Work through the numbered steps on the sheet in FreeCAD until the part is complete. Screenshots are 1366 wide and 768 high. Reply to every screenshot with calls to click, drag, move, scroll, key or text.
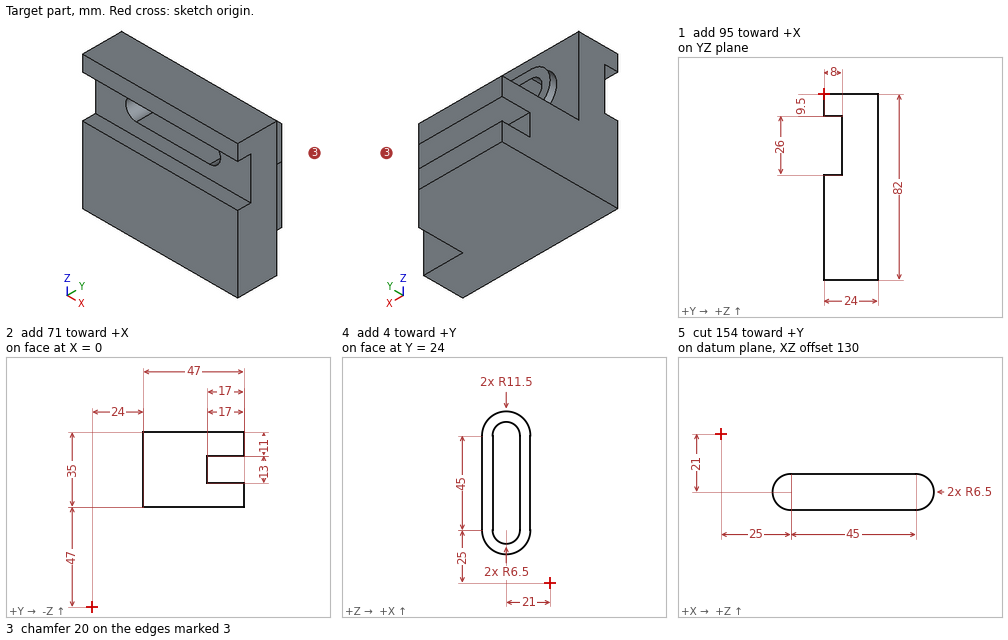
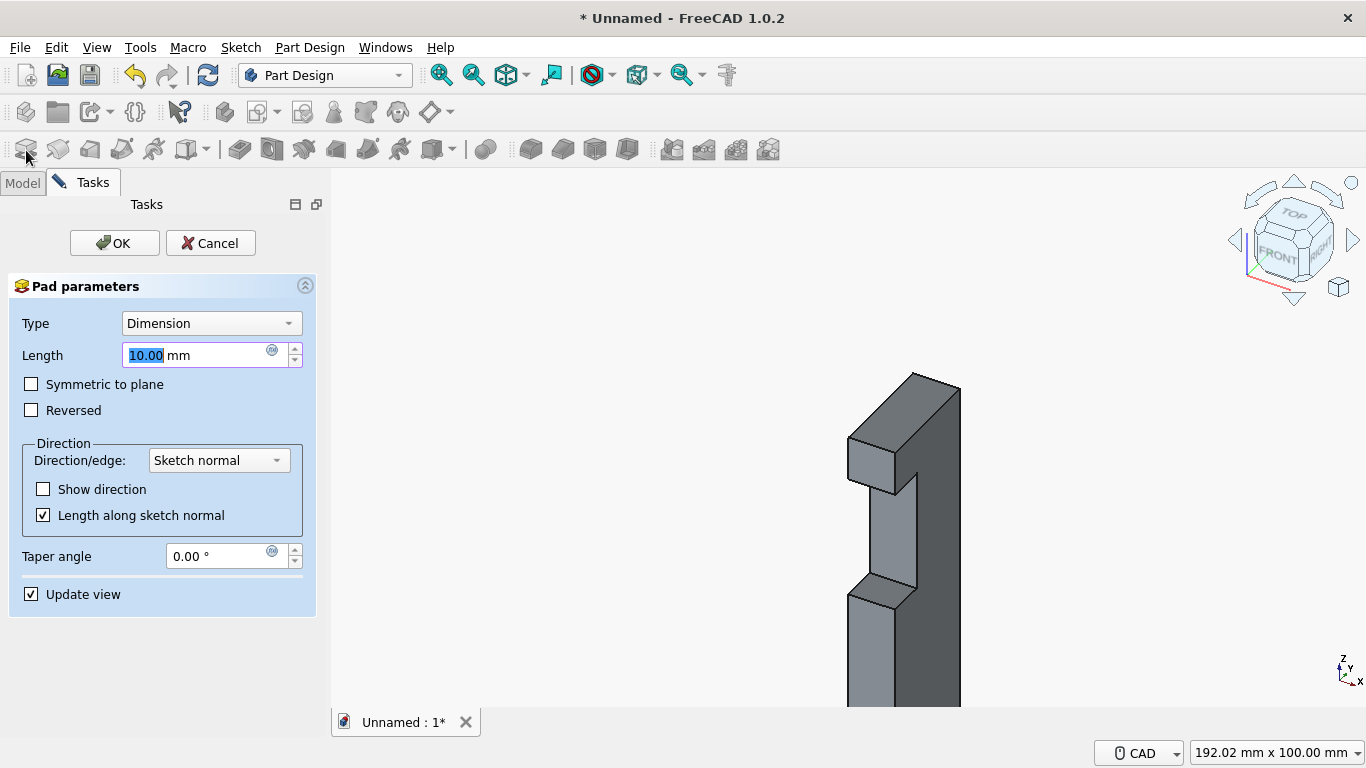
text(95)
key(Tab)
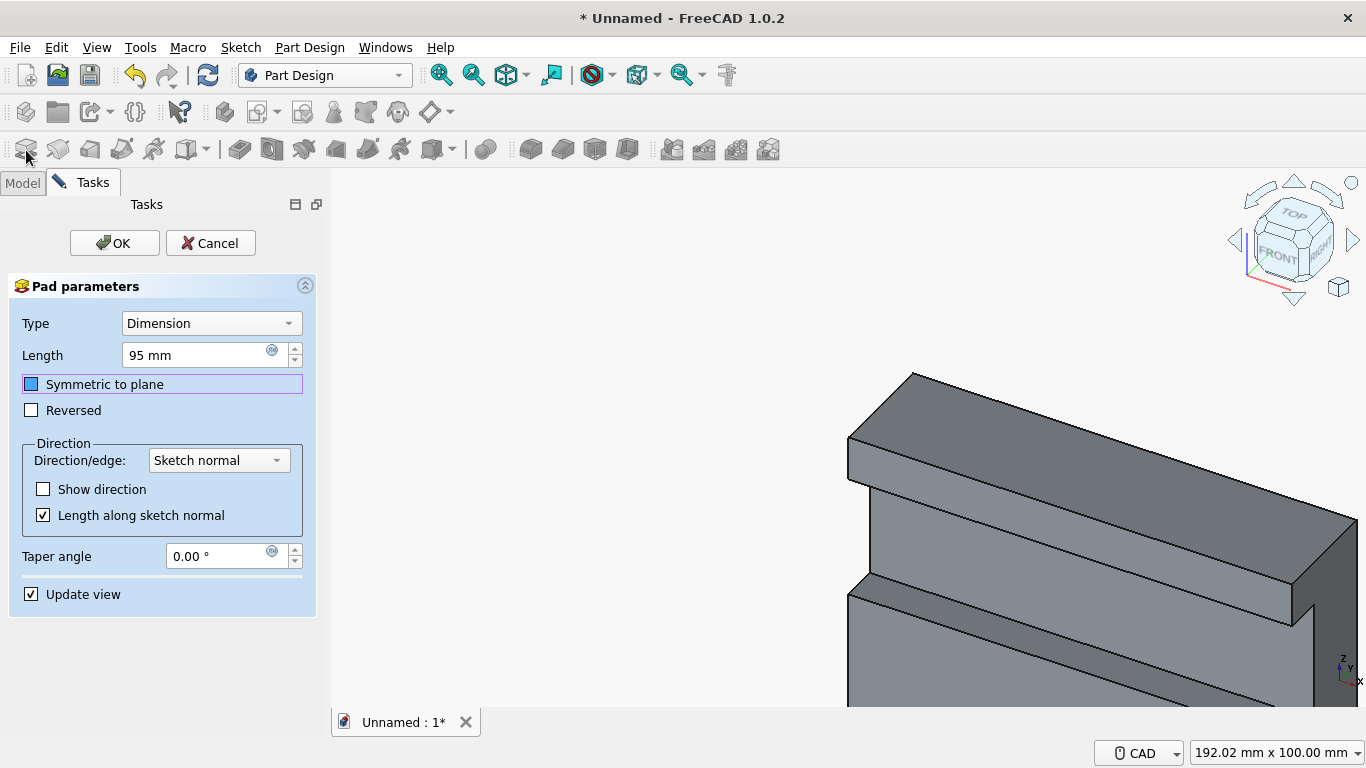
click(115, 243)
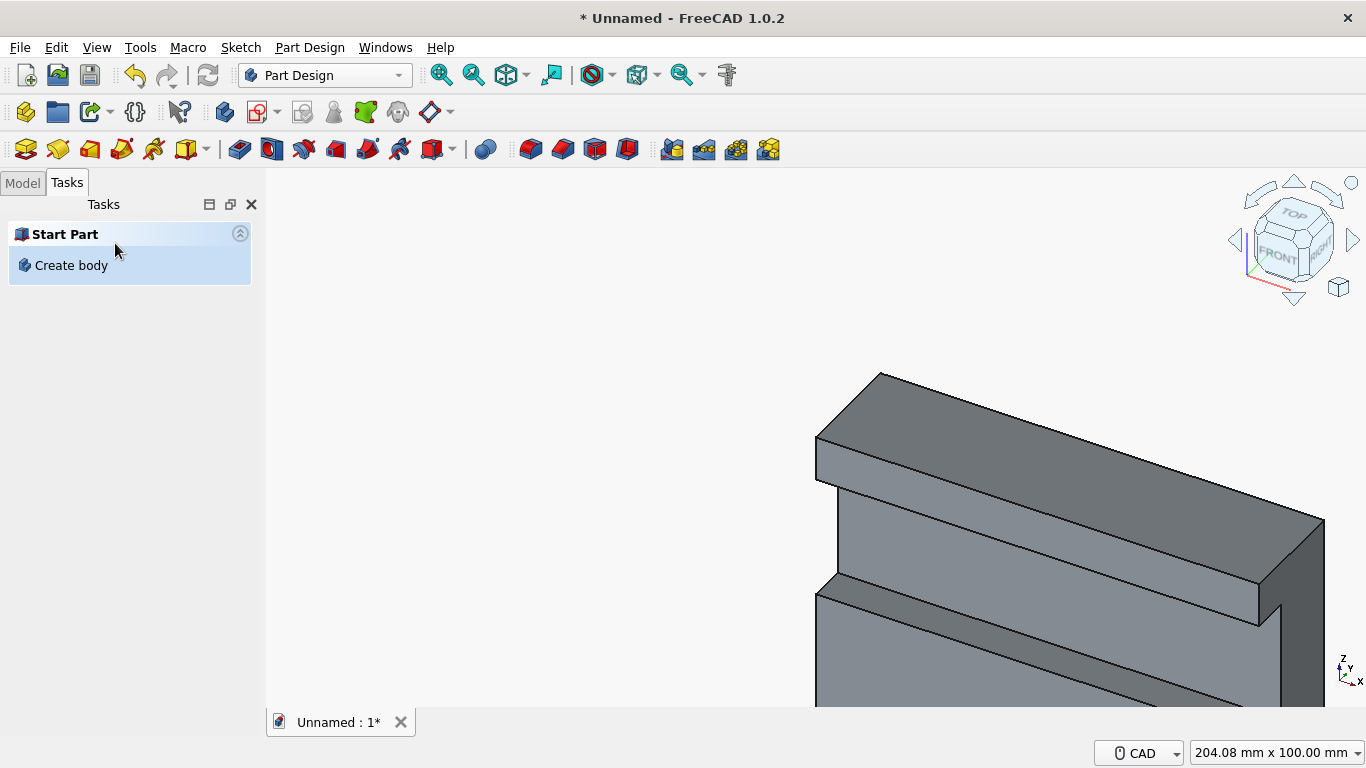
click(442, 76)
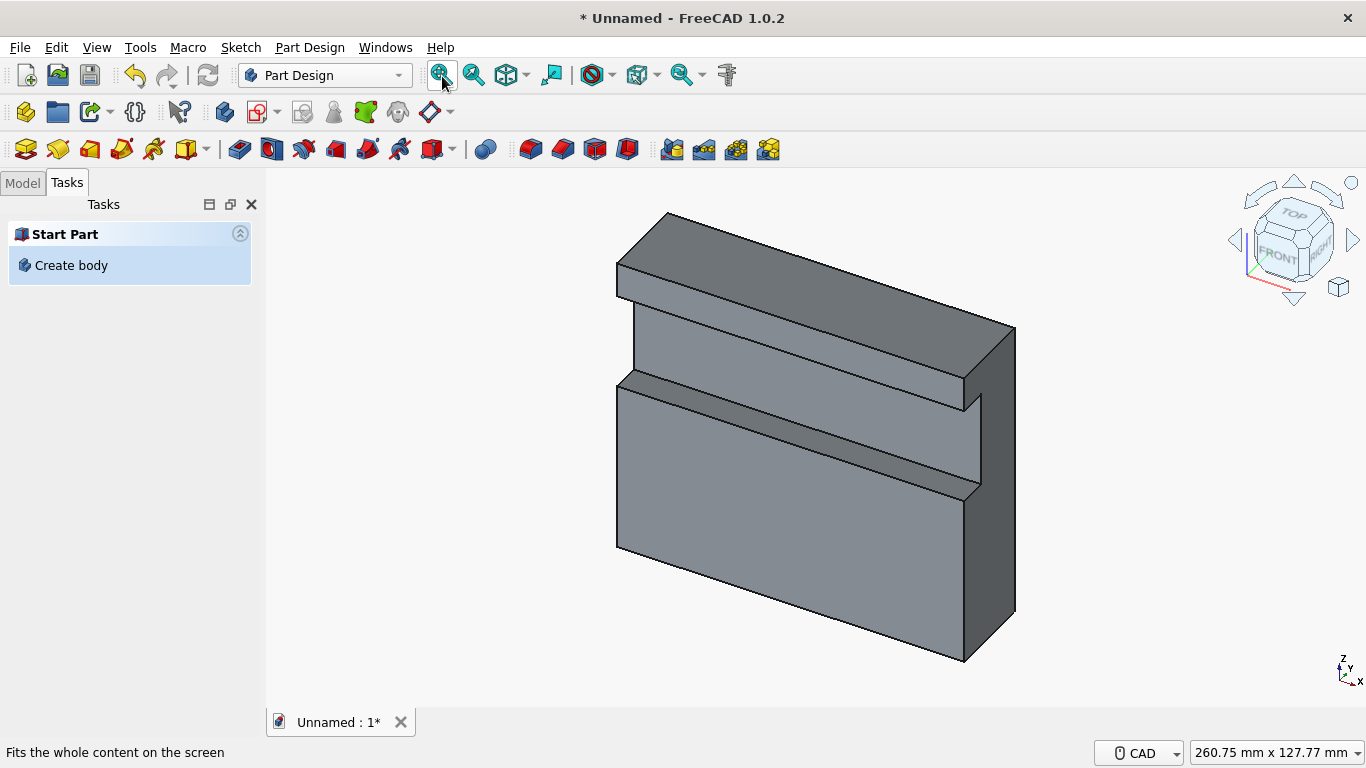
key(6)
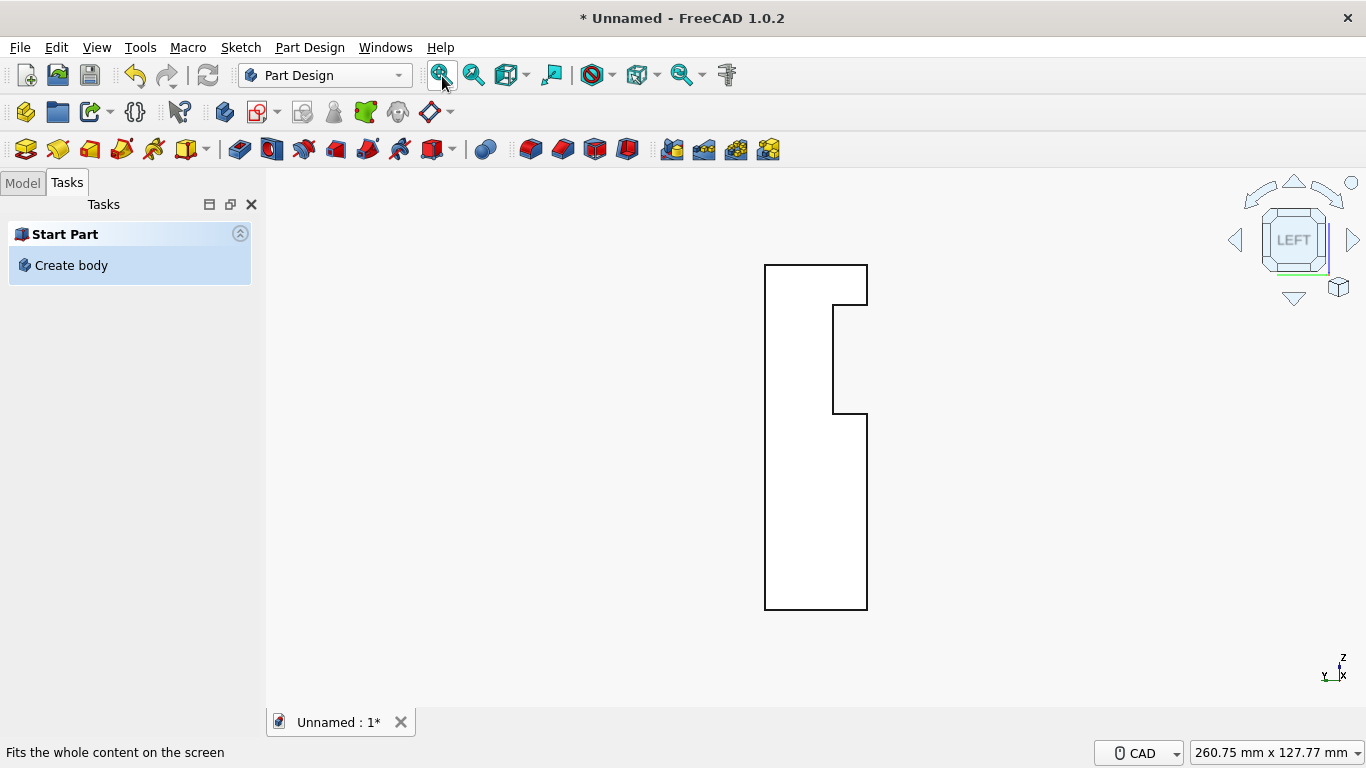
click(816, 535)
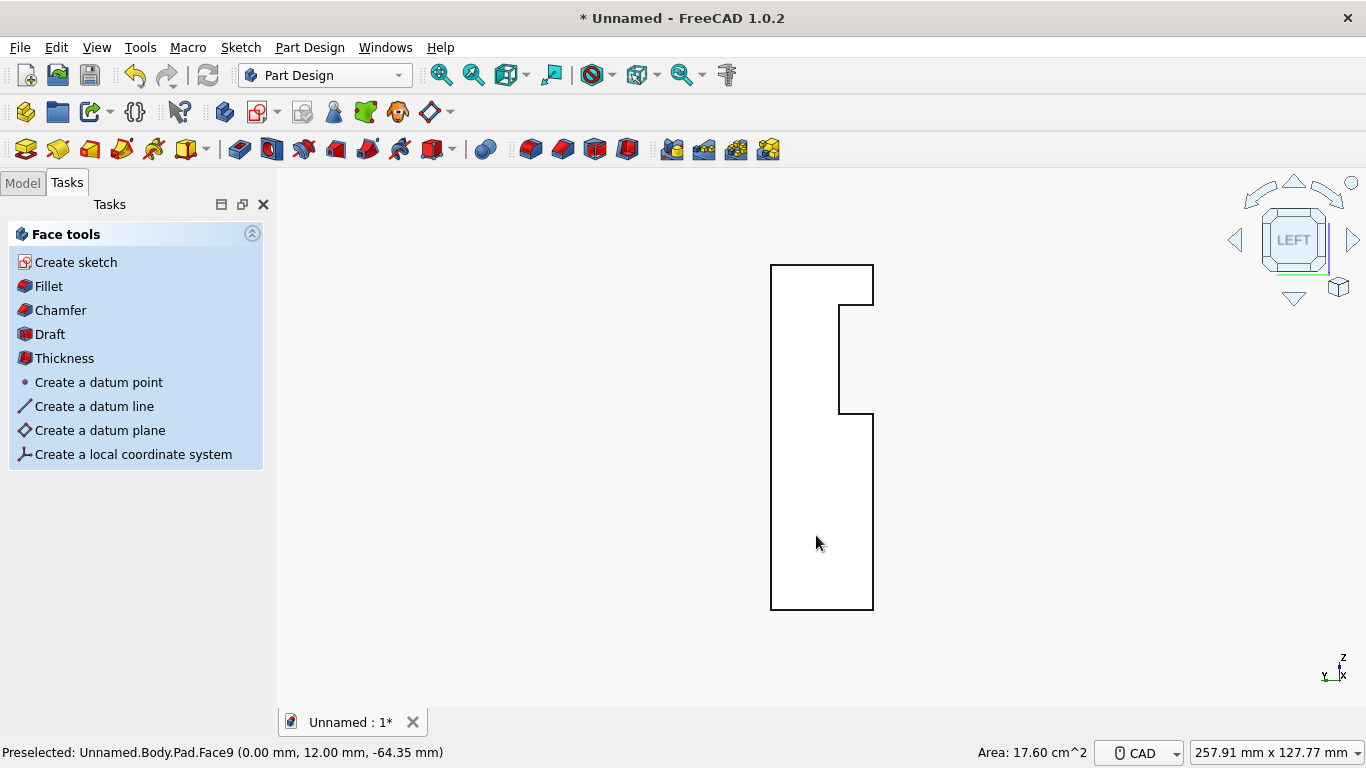
click(258, 112)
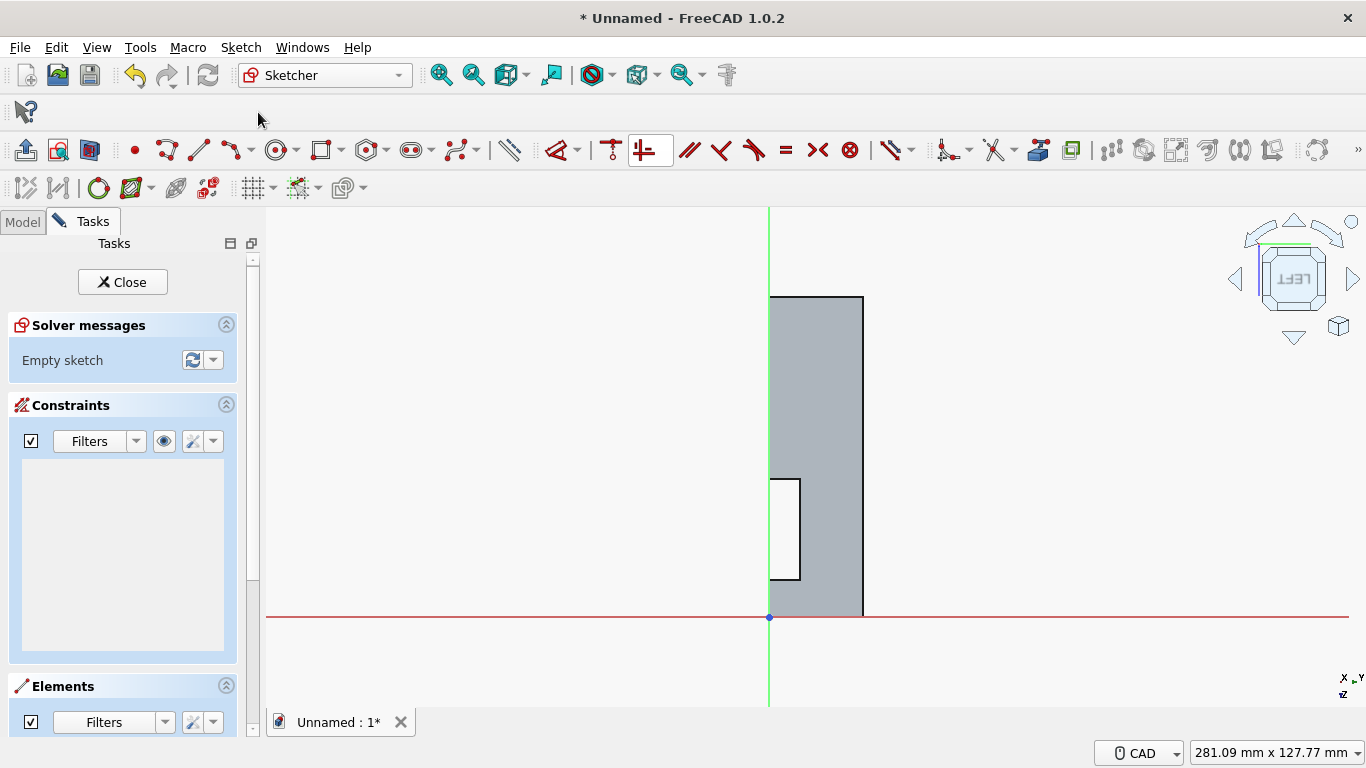
click(168, 150)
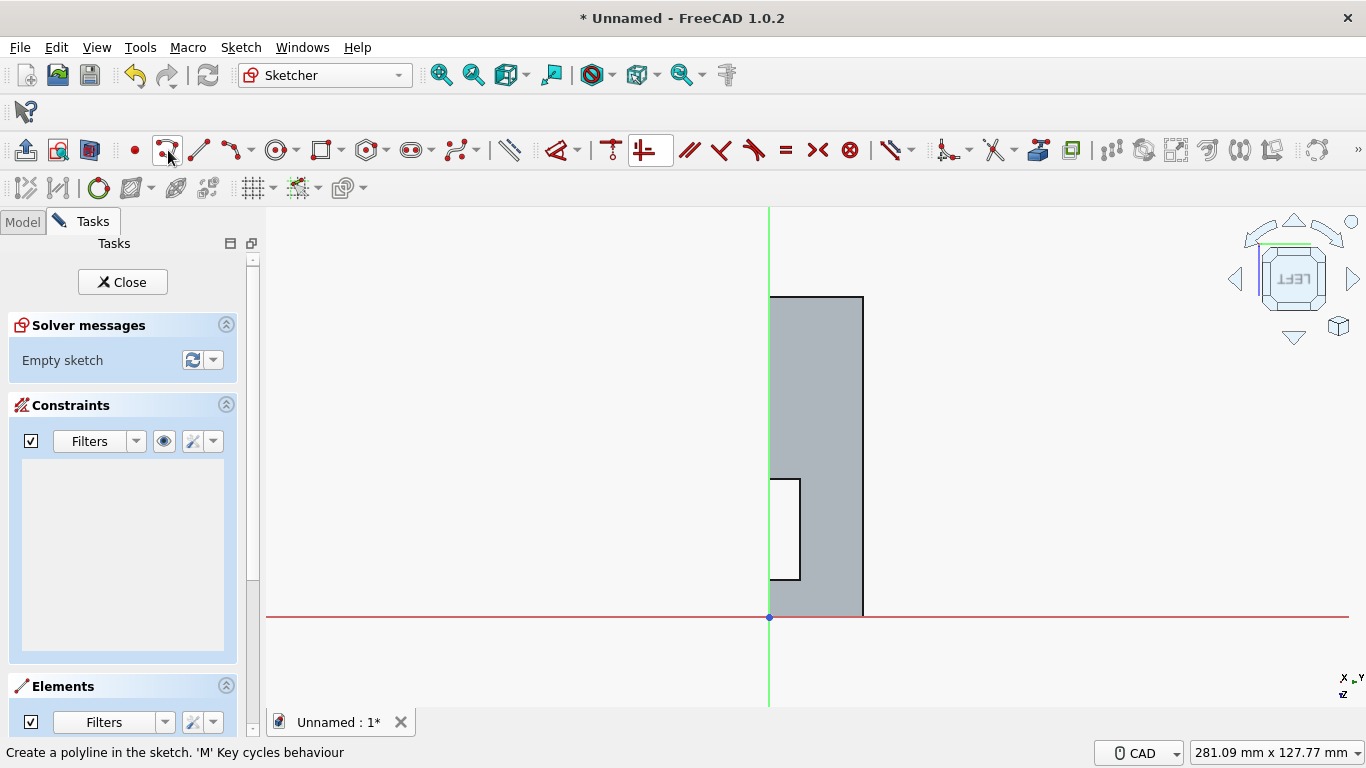
click(863, 434)
click(863, 297)
click(1047, 297)
click(1047, 340)
click(980, 340)
click(980, 390)
click(1047, 390)
click(1047, 434)
click(863, 435)
key(Escape)
key(Escape)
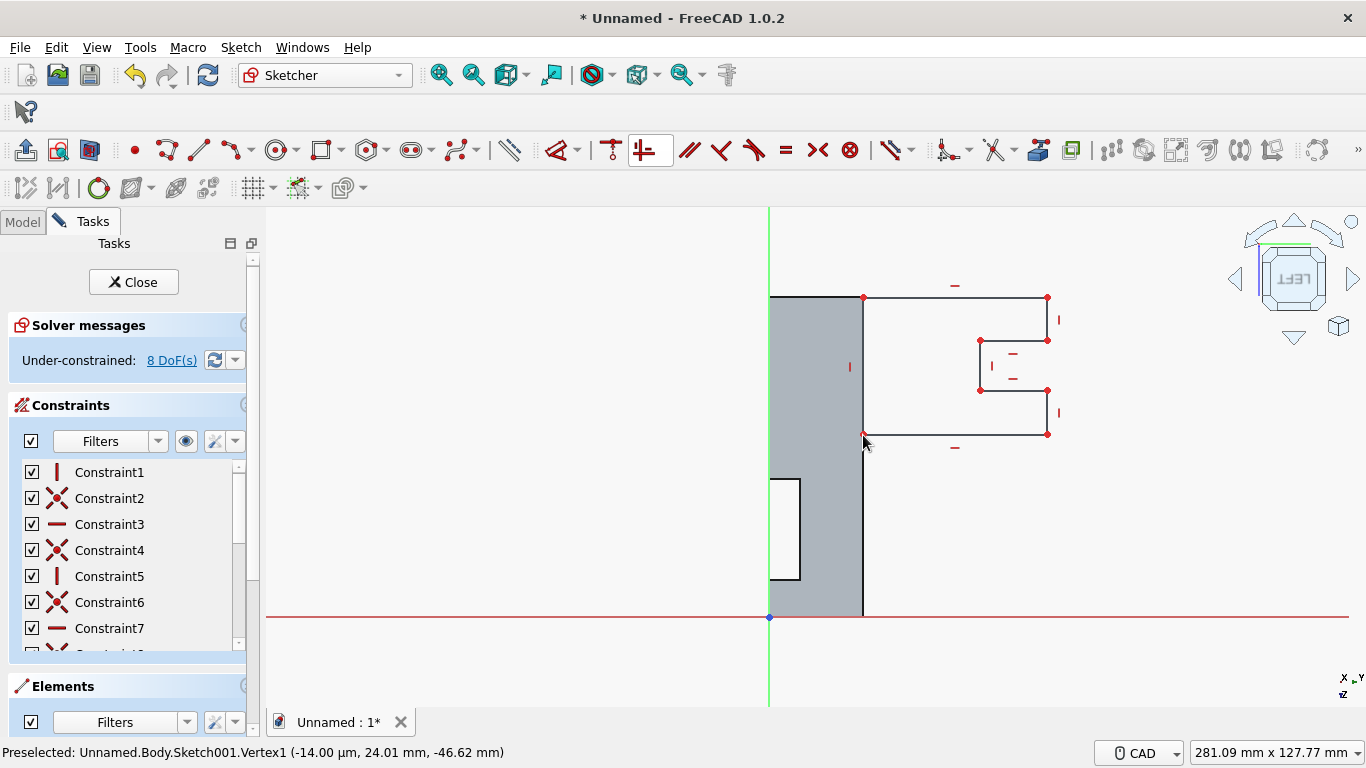
click(556, 150)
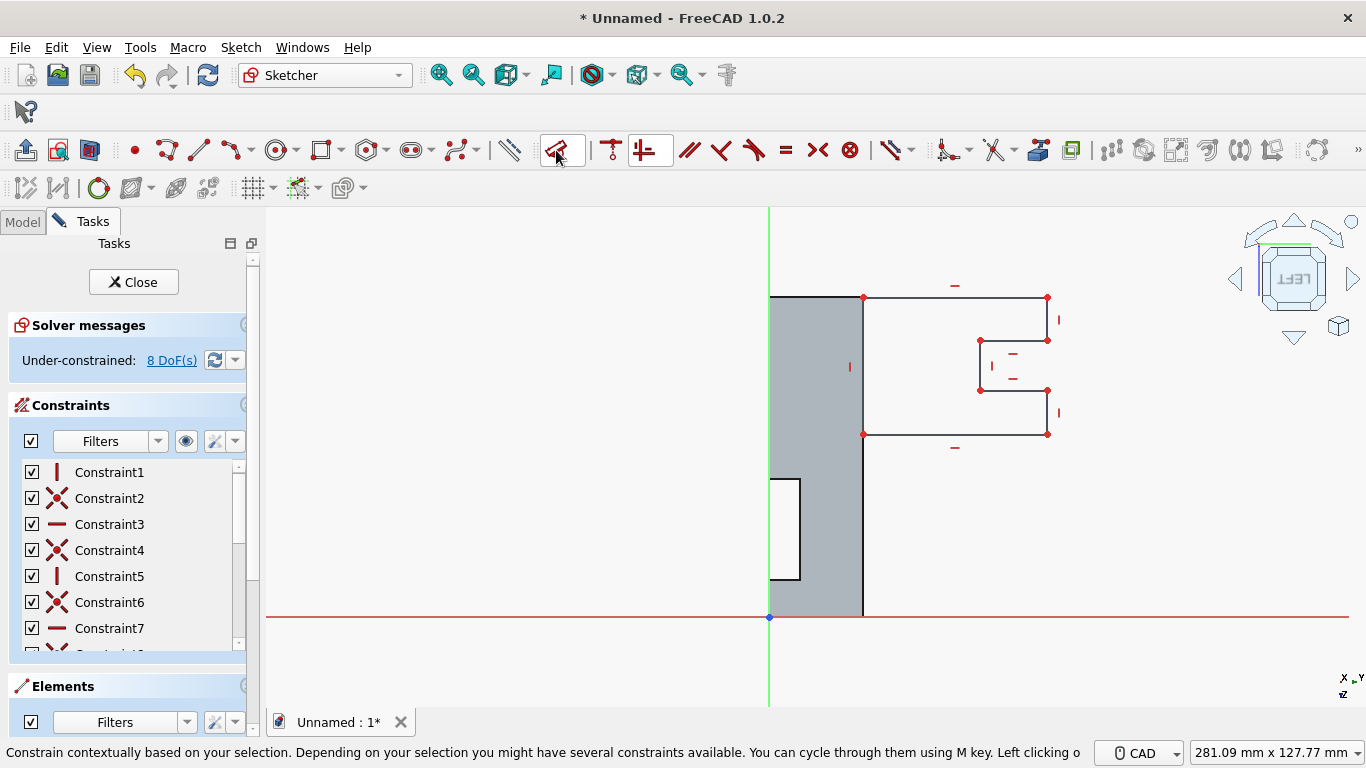
click(863, 394)
click(829, 366)